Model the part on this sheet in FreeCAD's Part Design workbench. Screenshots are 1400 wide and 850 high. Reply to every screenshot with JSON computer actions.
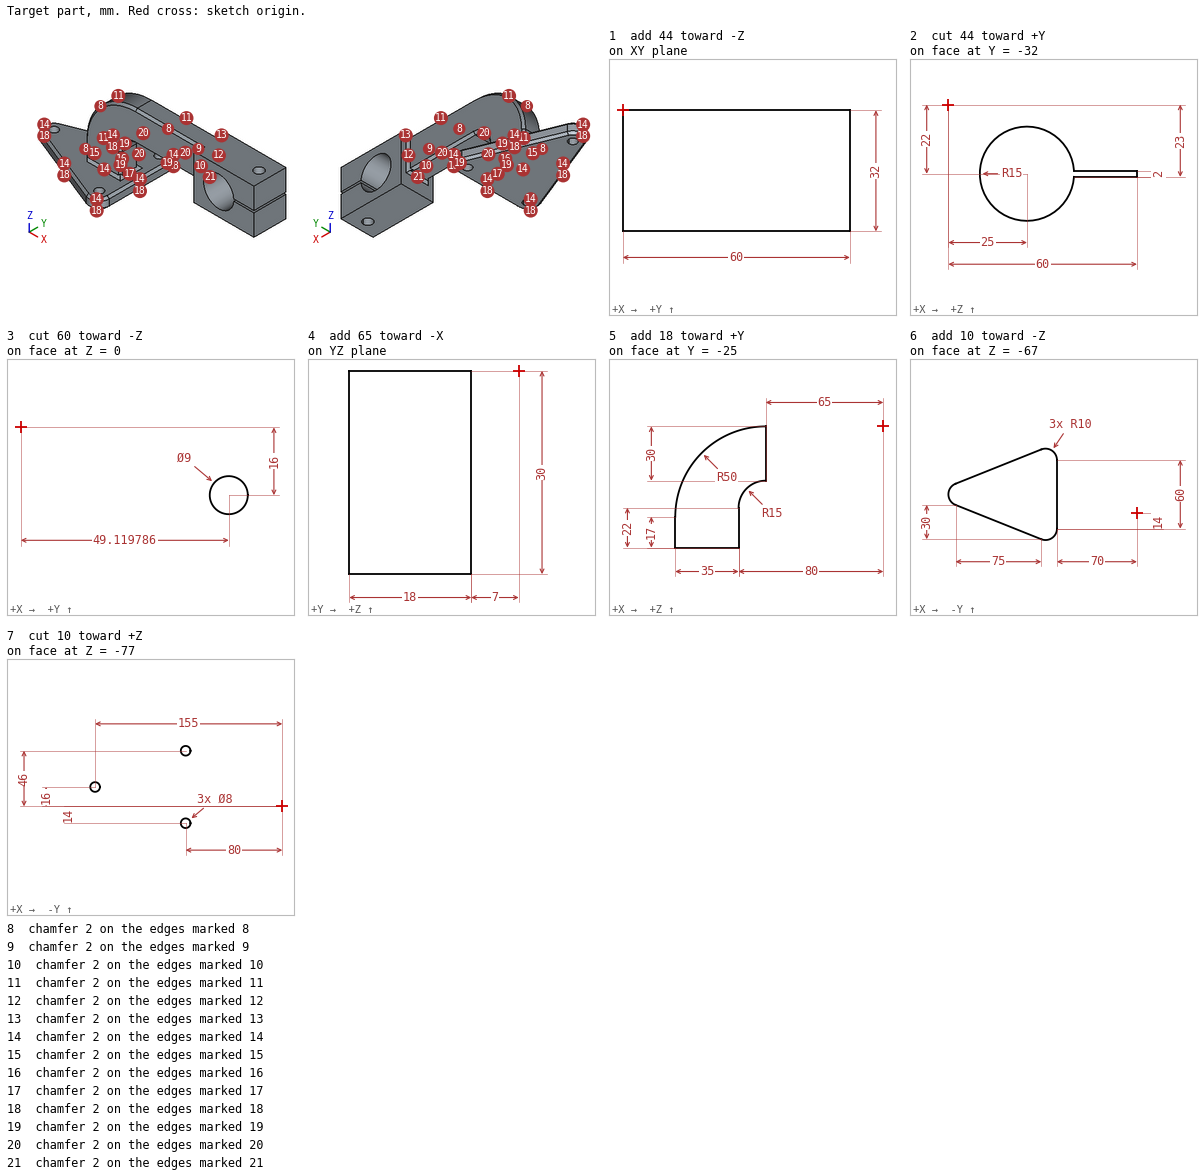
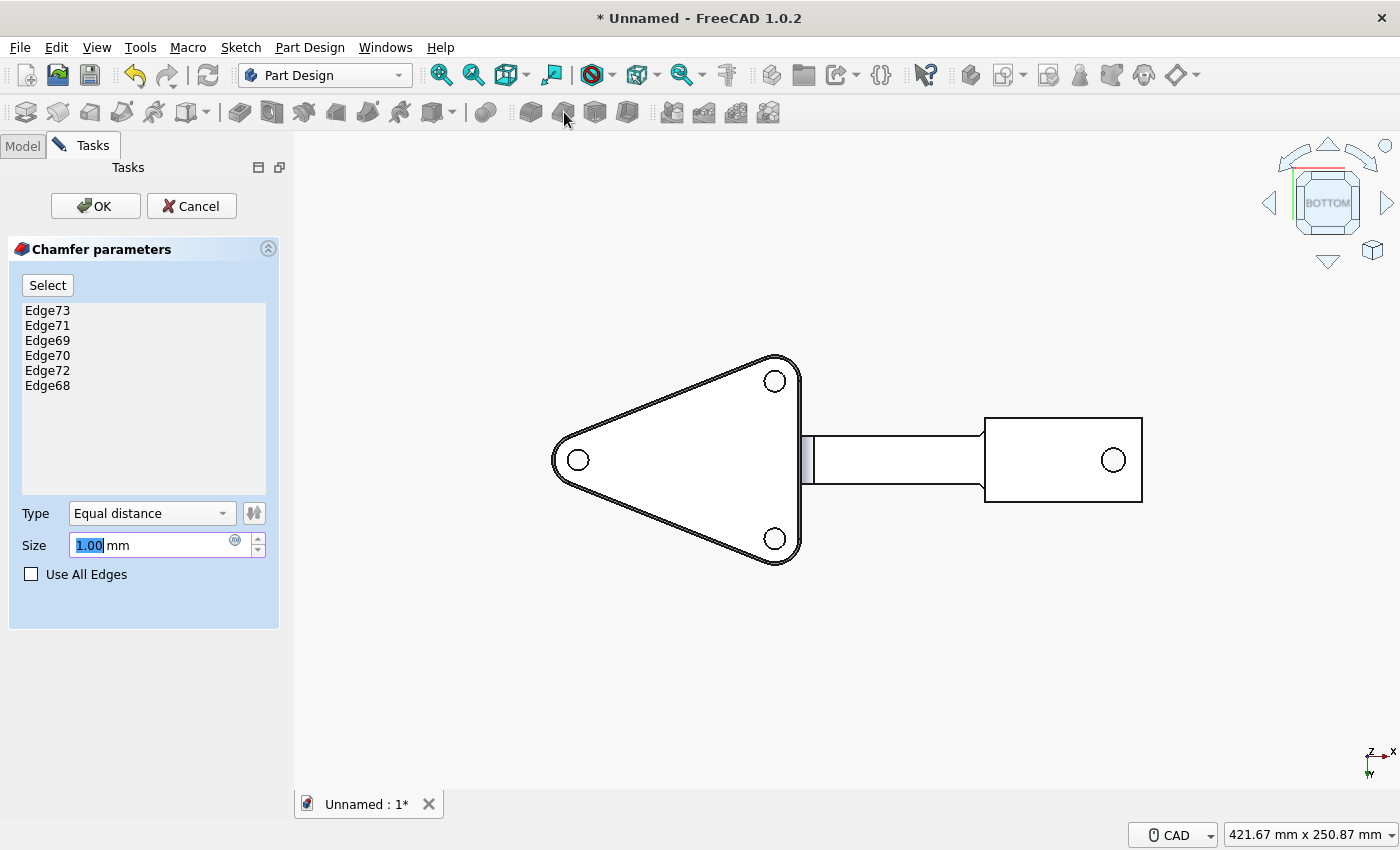
{"action": "type", "text": "2"}
{"action": "key", "text": "Tab"}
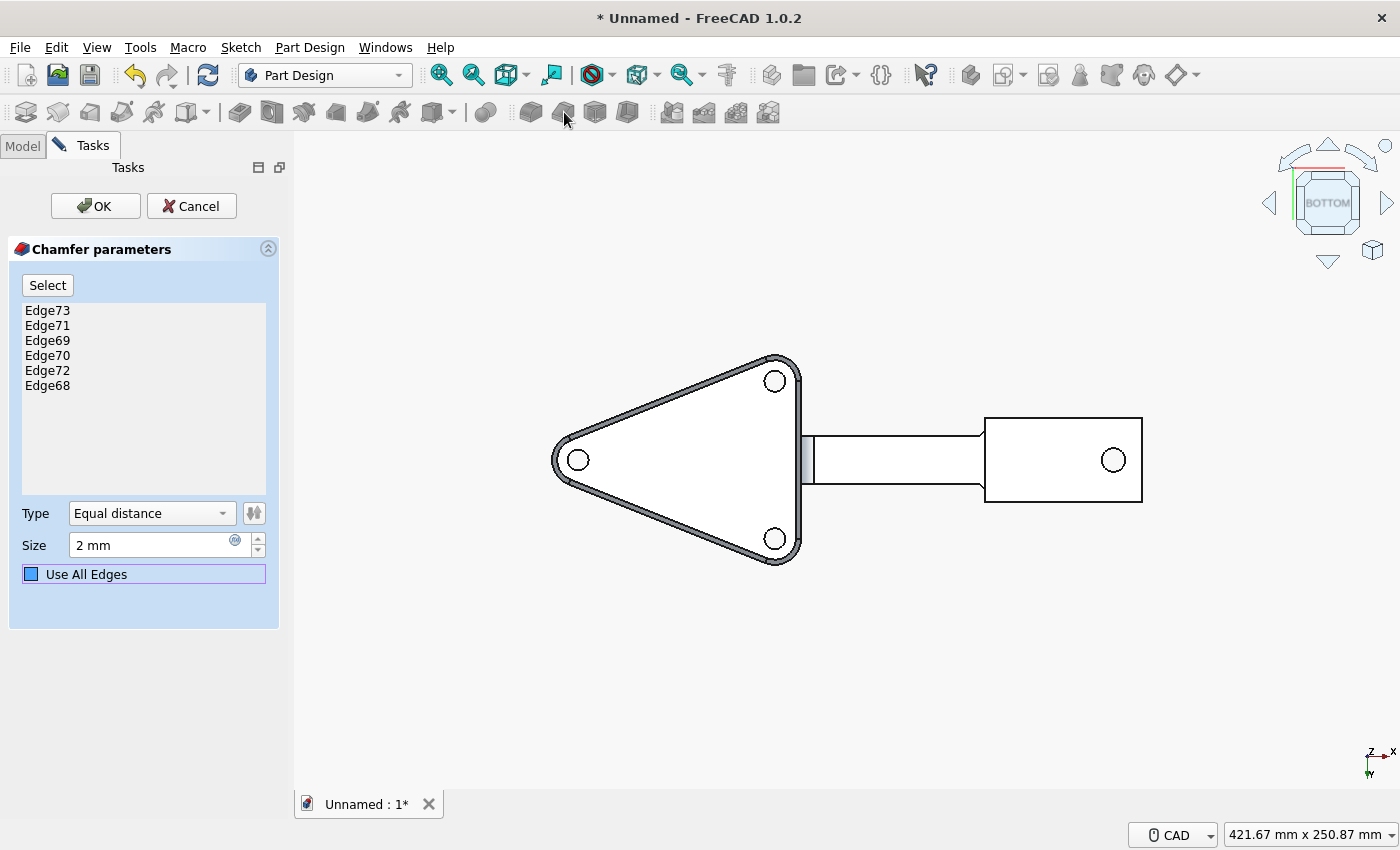
{"action": "left_click", "coordinate": [96, 206]}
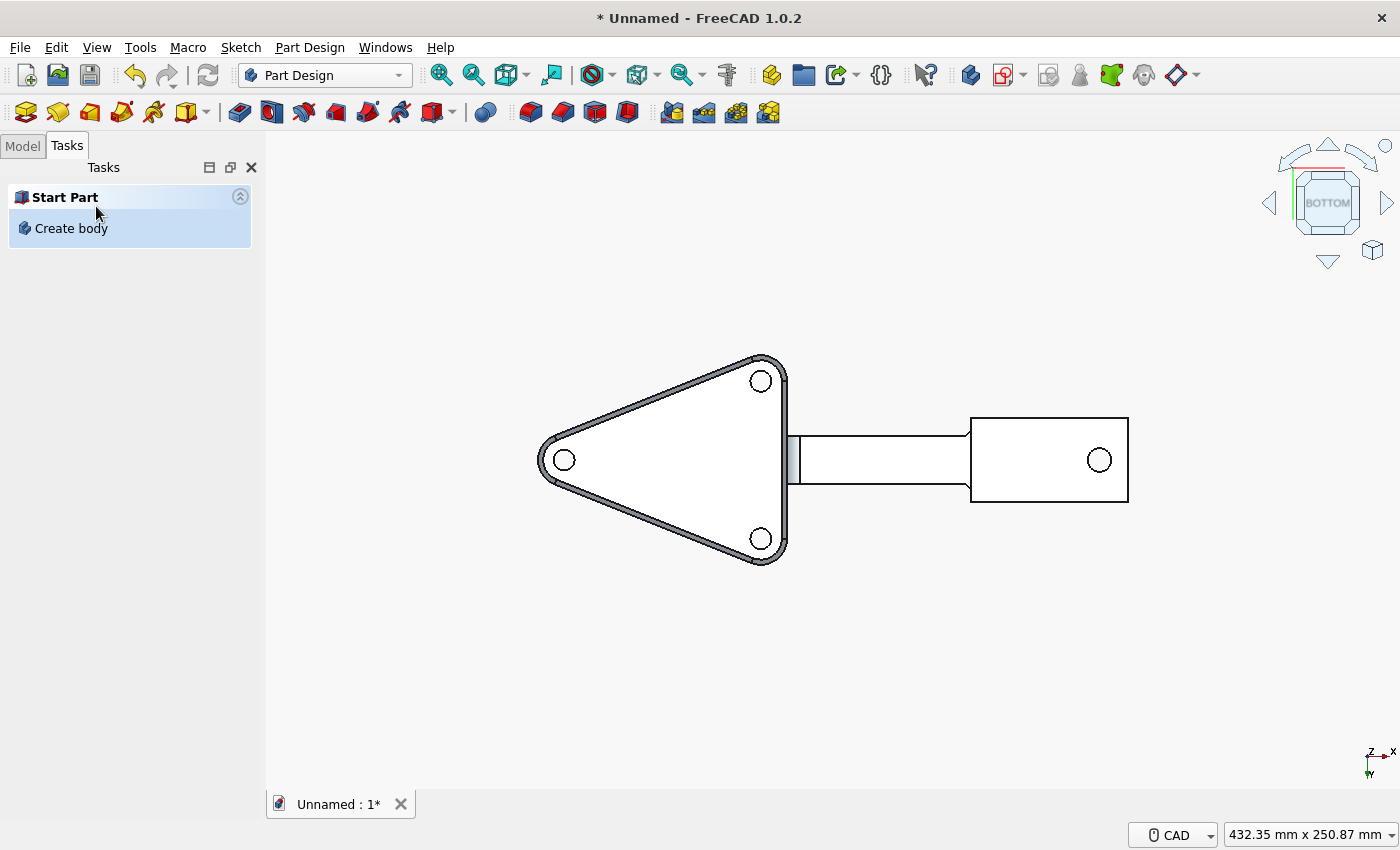
{"action": "left_click", "coordinate": [883, 435]}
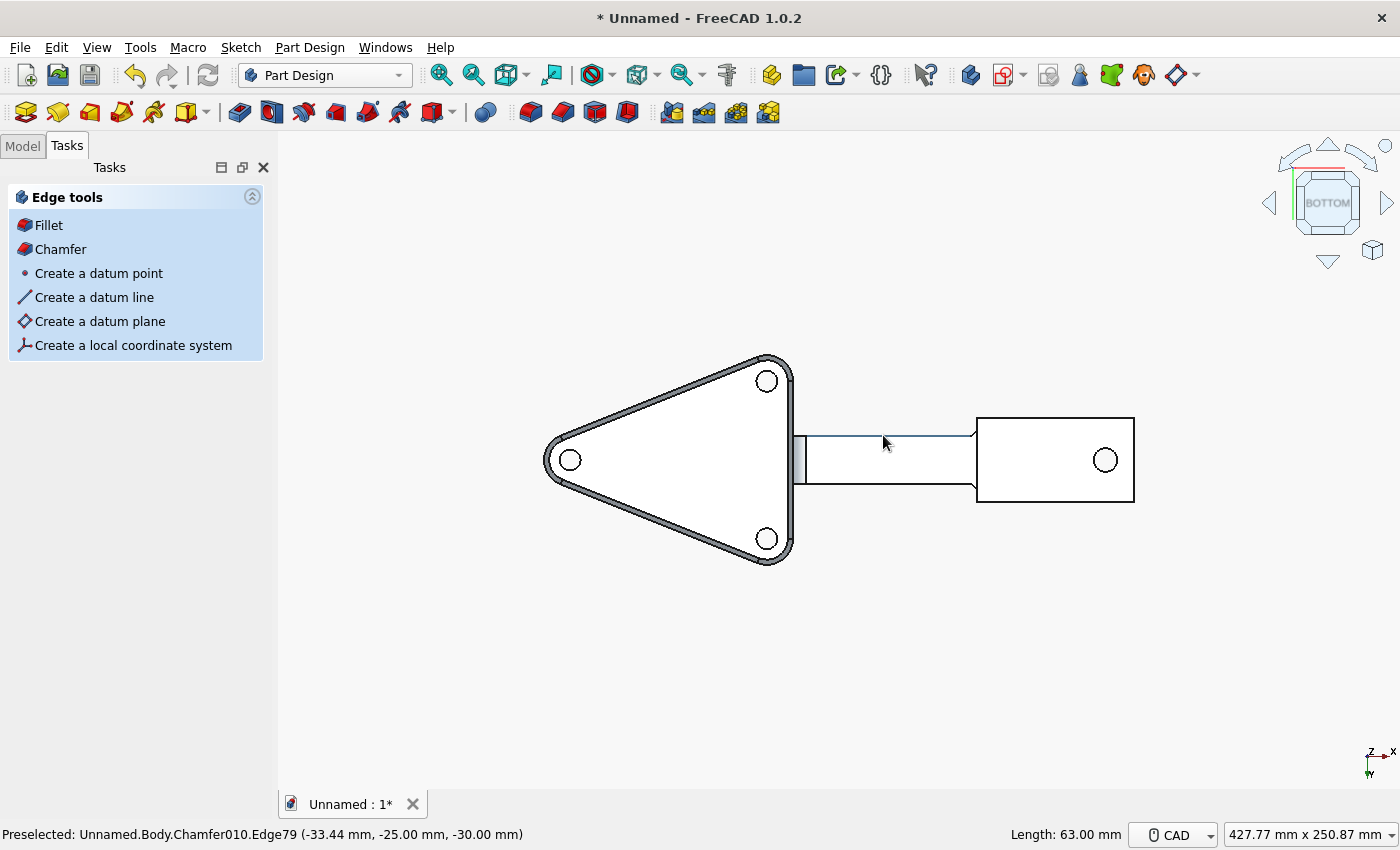
{"action": "left_click", "coordinate": [804, 435], "text": "ctrl"}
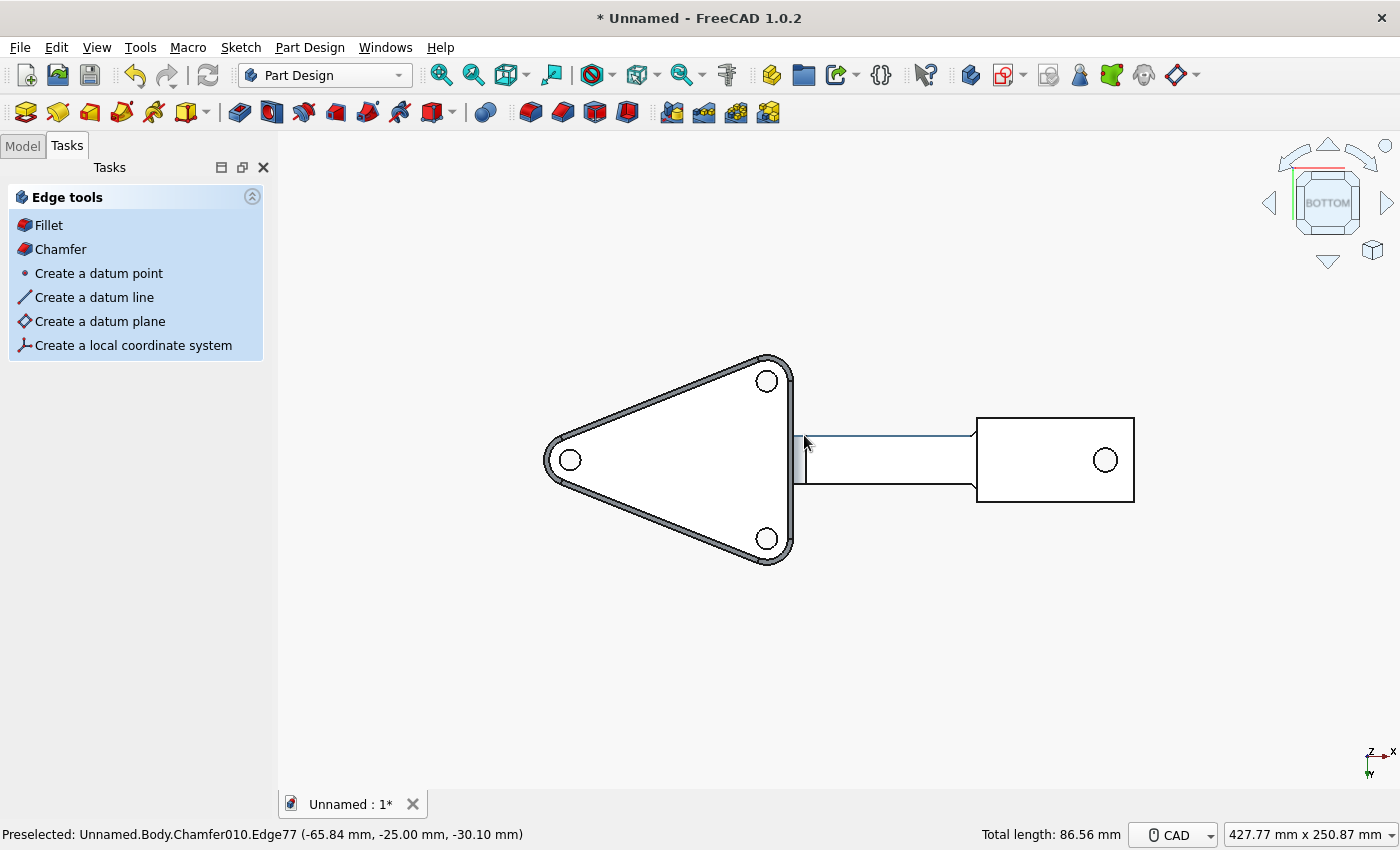
{"action": "key", "text": "0"}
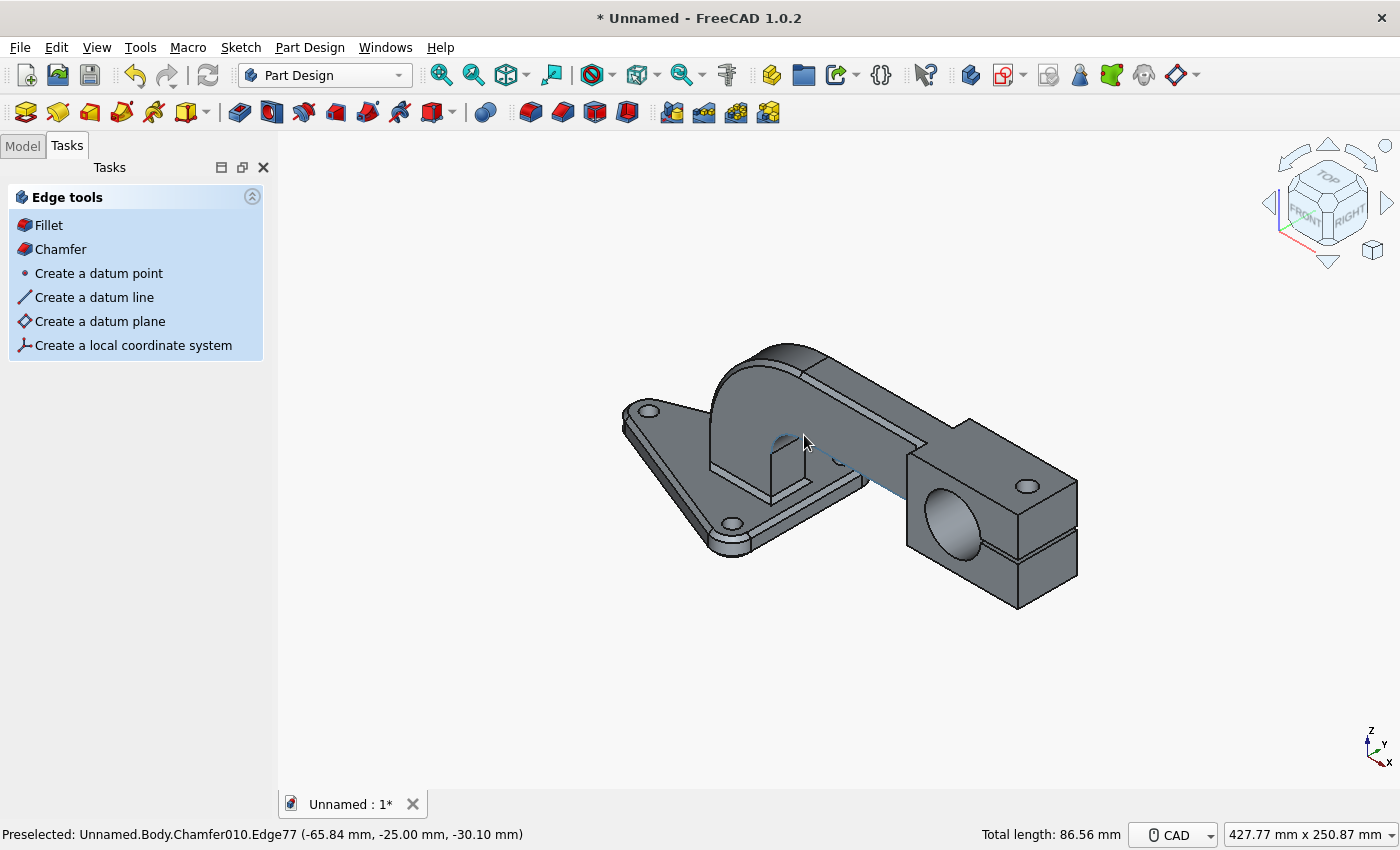
{"action": "left_click", "coordinate": [771, 475], "text": "ctrl"}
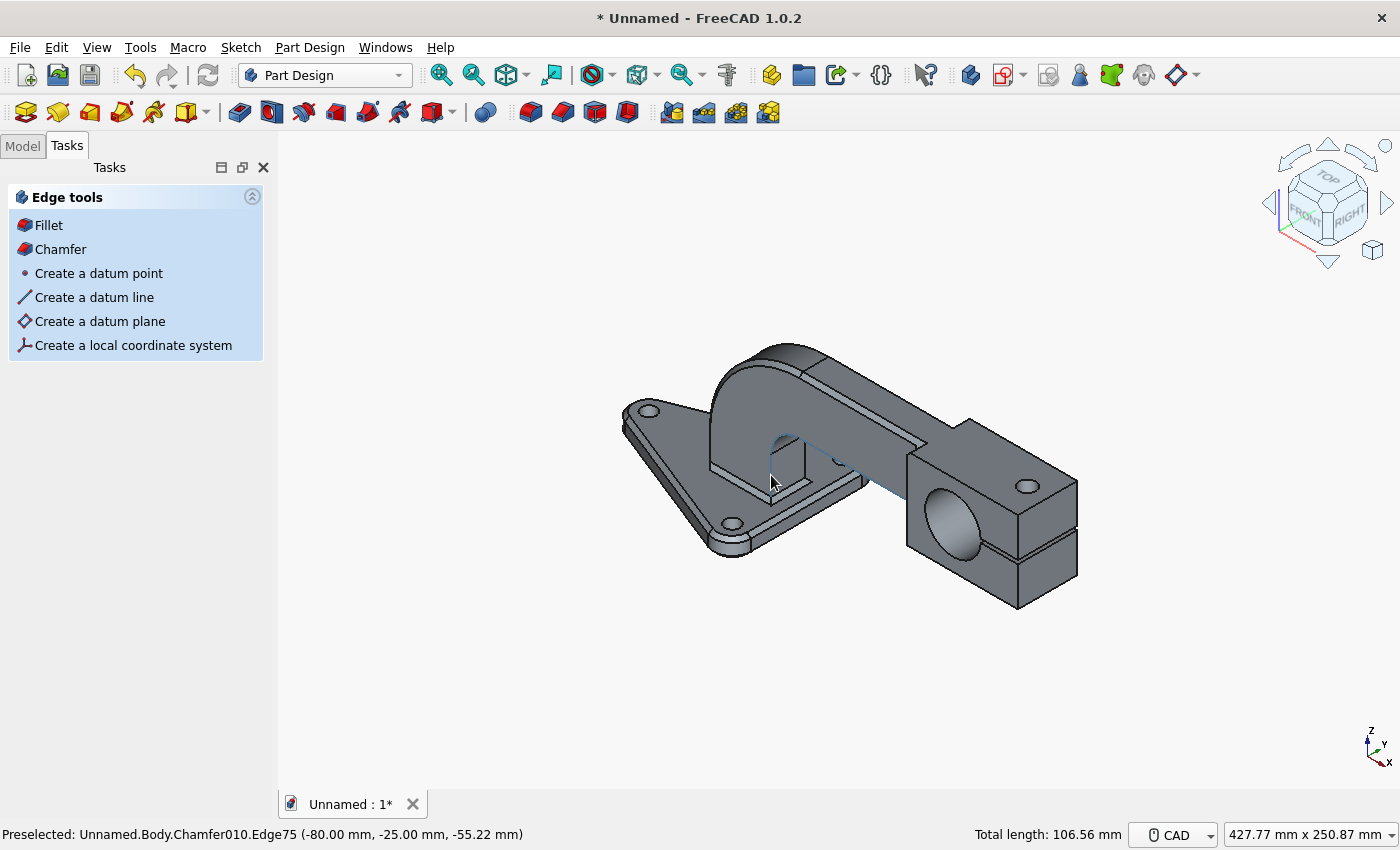
{"action": "left_click", "coordinate": [564, 112]}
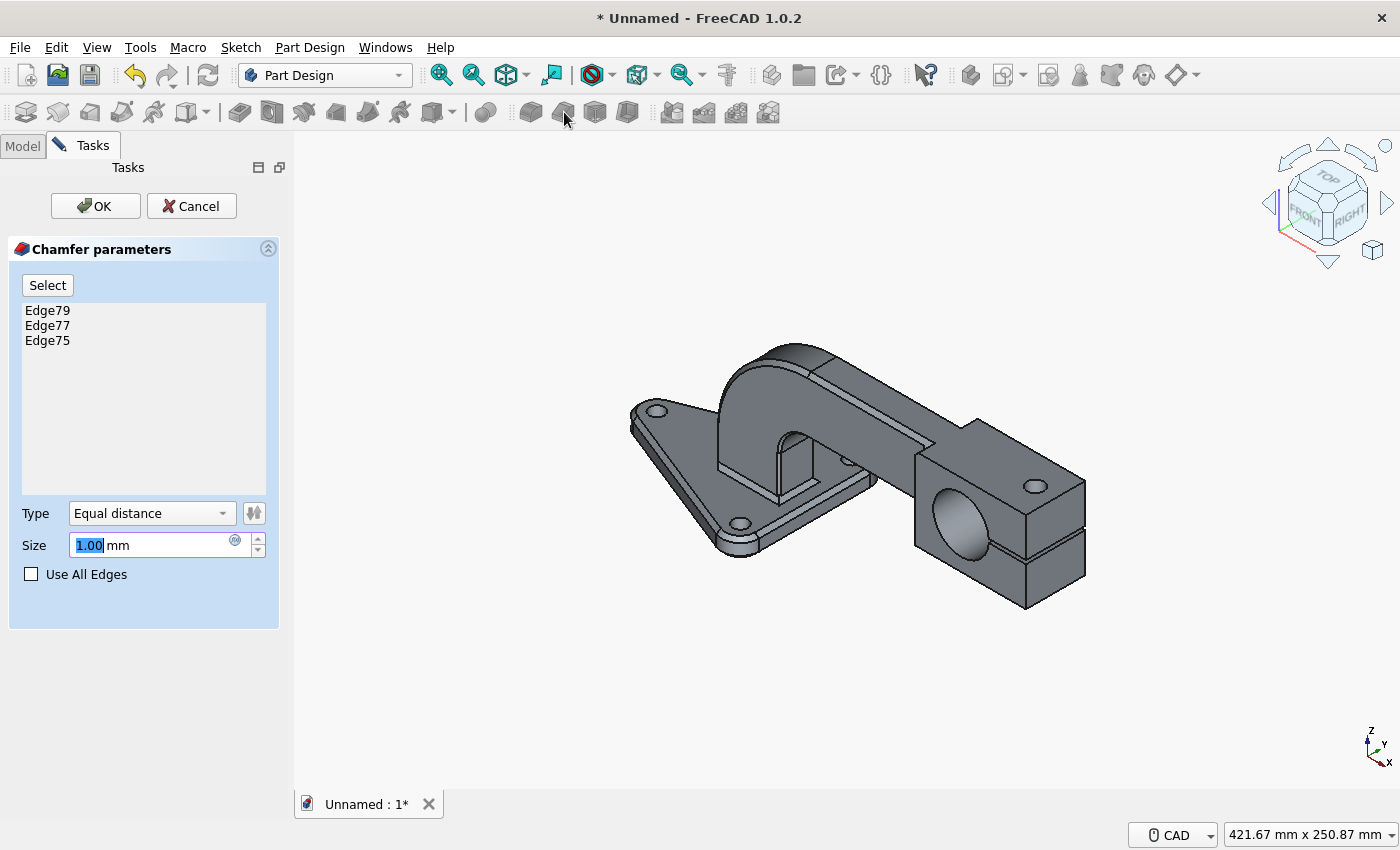
{"action": "type", "text": "2"}
{"action": "key", "text": "Tab"}